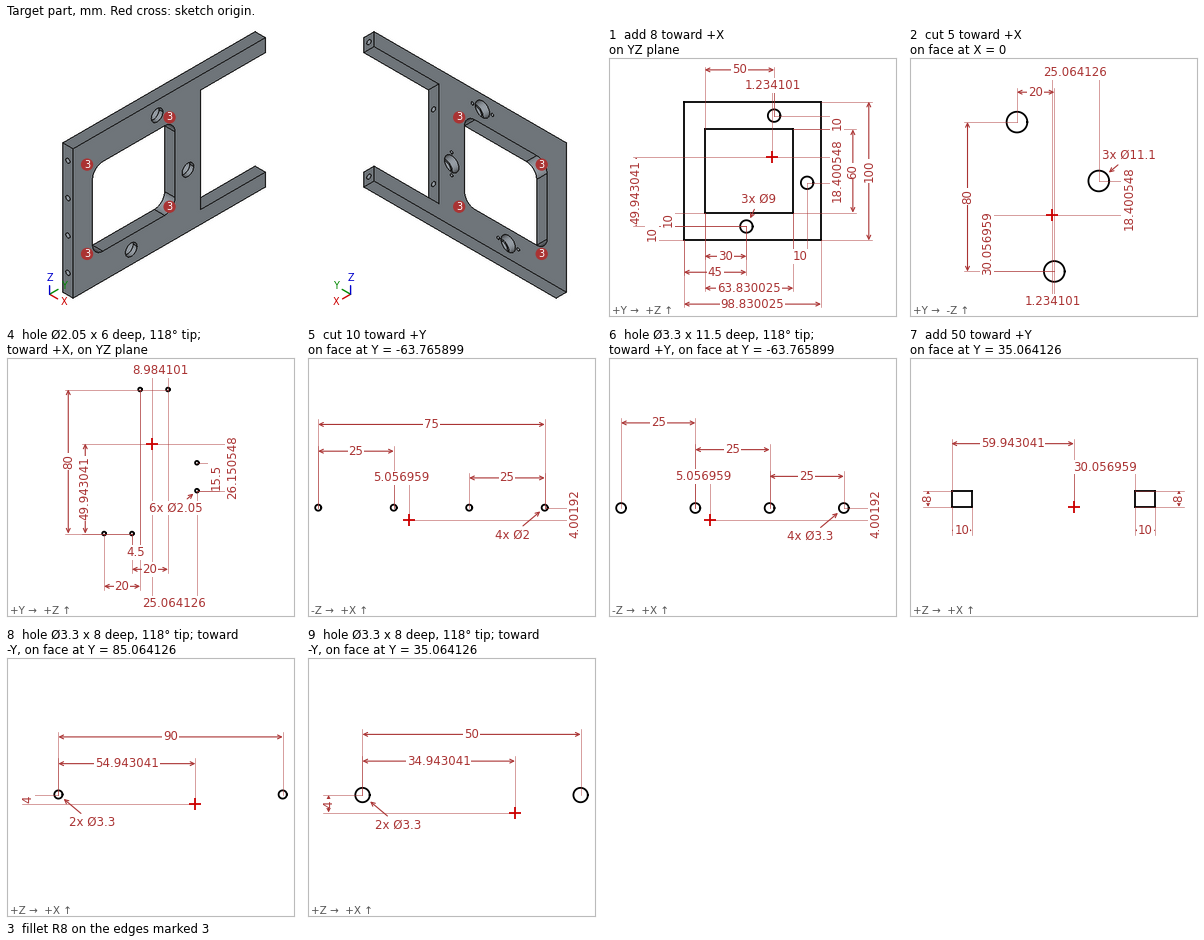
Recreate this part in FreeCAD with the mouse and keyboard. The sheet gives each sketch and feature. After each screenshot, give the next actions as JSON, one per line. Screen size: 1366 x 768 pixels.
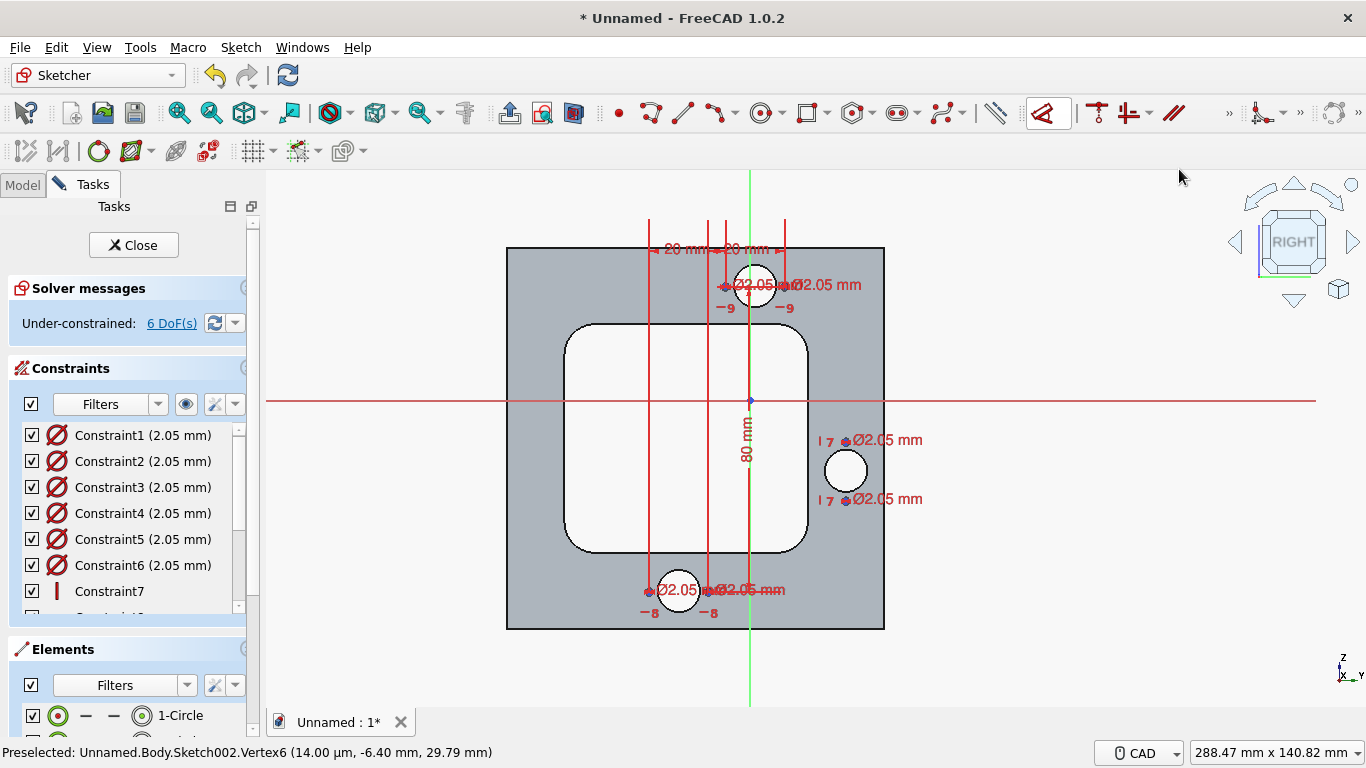
{"action": "scroll", "coordinate": [708, 592], "scroll_direction": "up", "scroll_amount": 5}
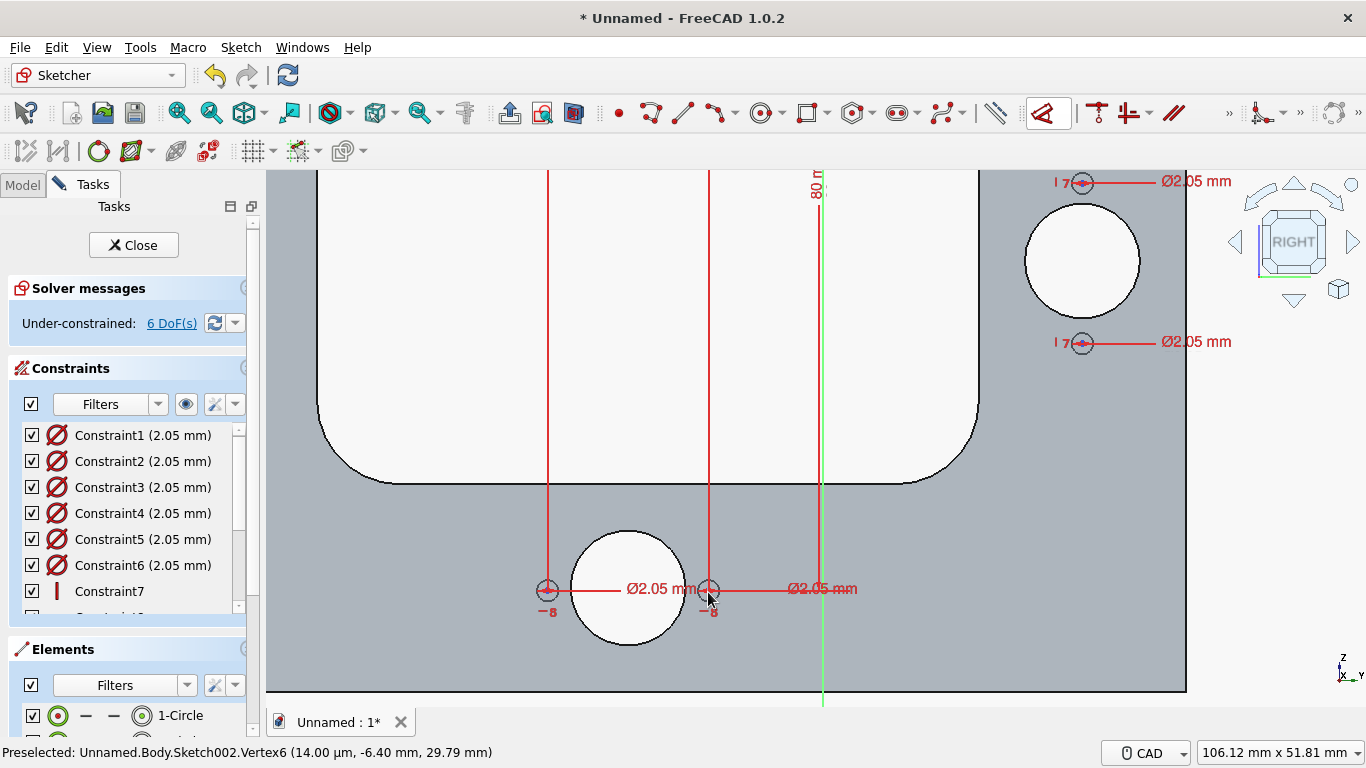
{"action": "left_click", "coordinate": [709, 591]}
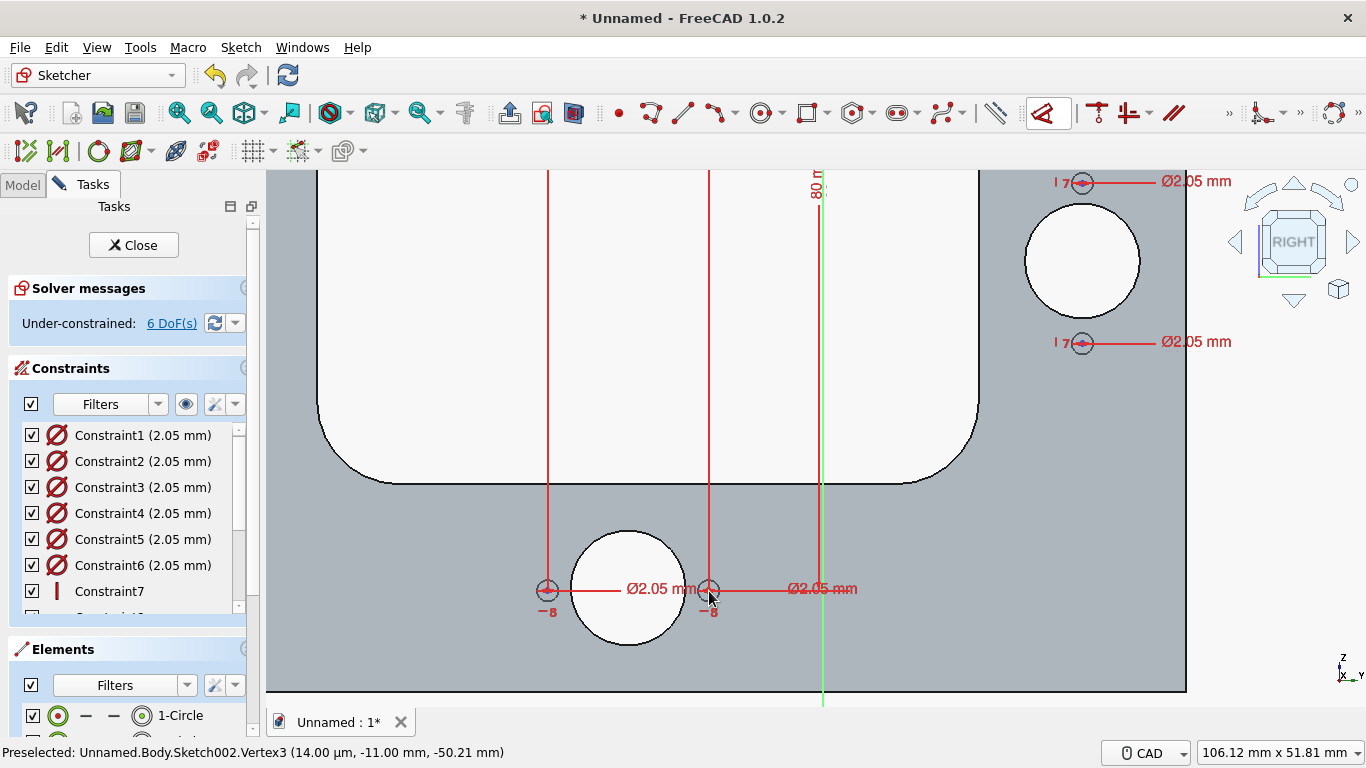
{"action": "scroll", "coordinate": [708, 593], "scroll_direction": "down", "scroll_amount": 5}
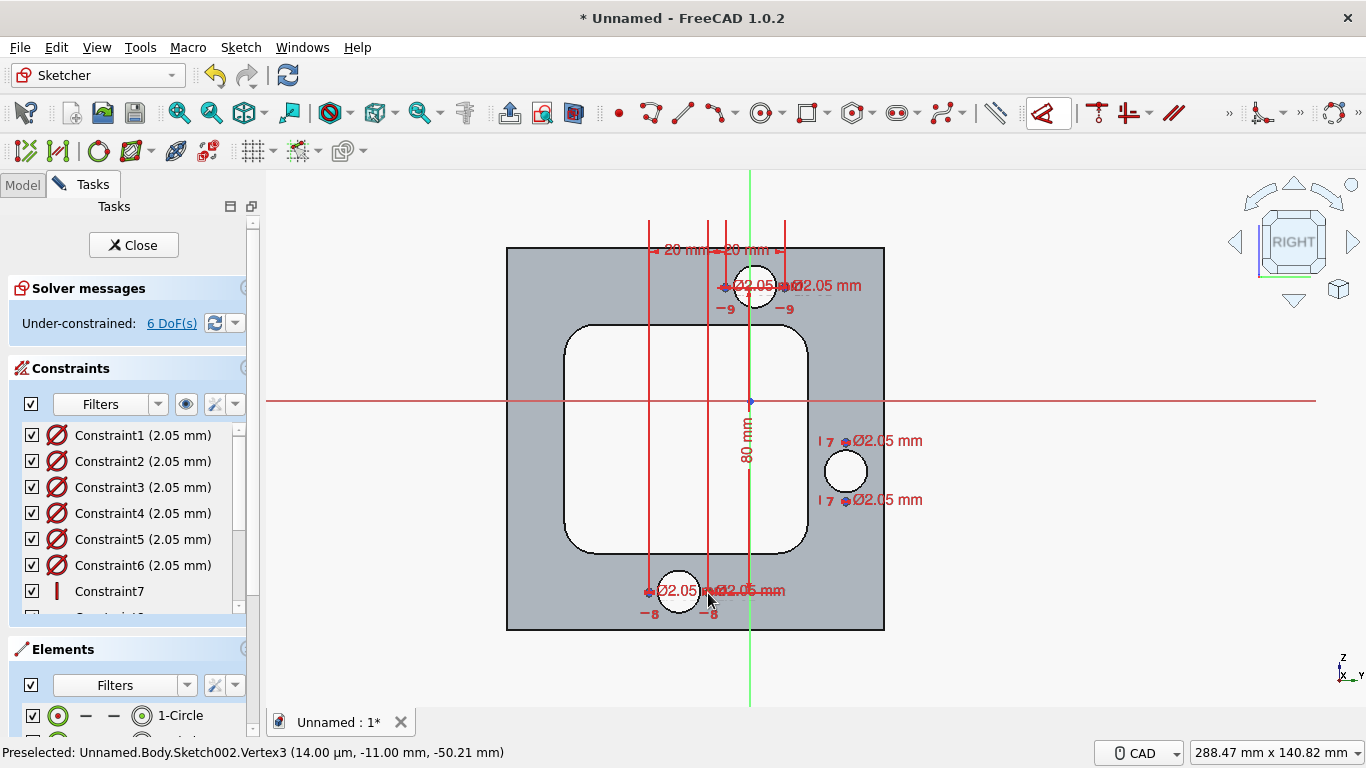
{"action": "scroll", "coordinate": [726, 288], "scroll_direction": "up", "scroll_amount": 5}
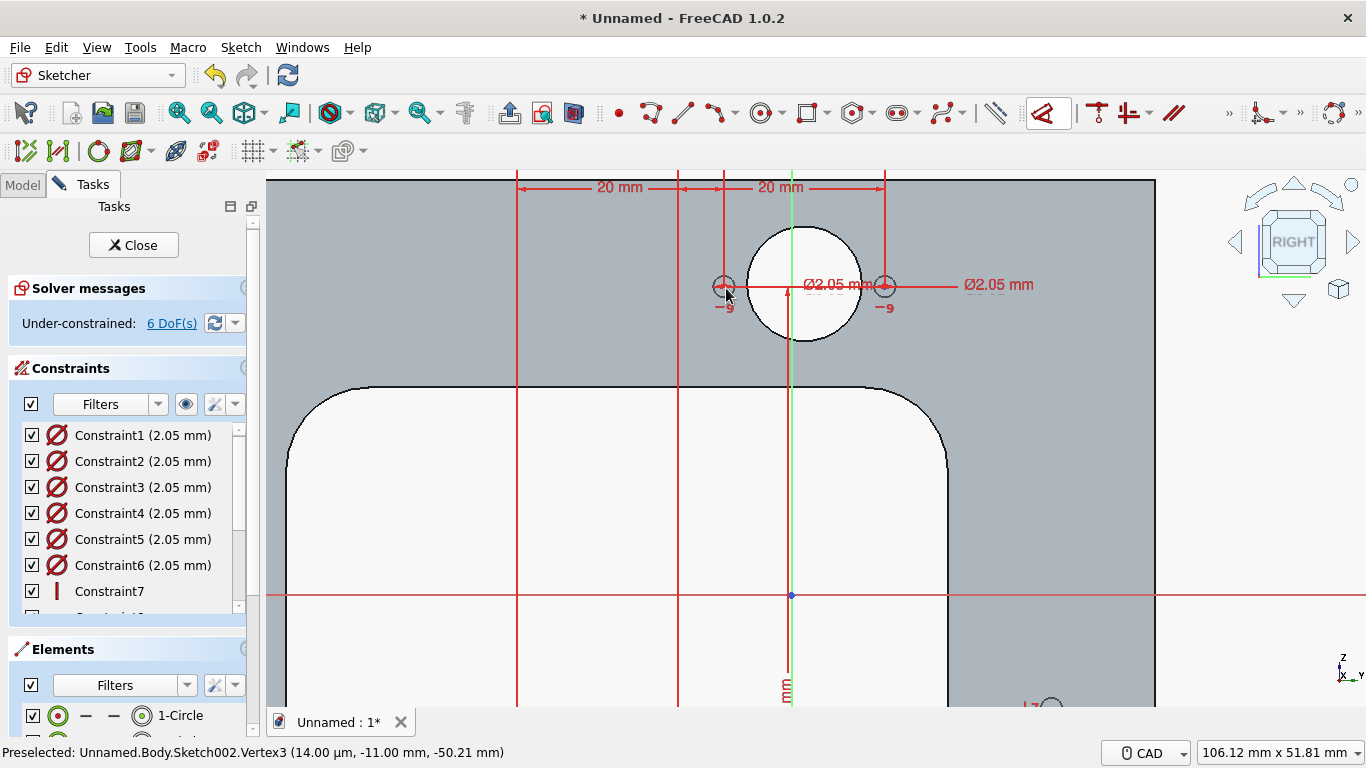
{"action": "left_click", "coordinate": [724, 287]}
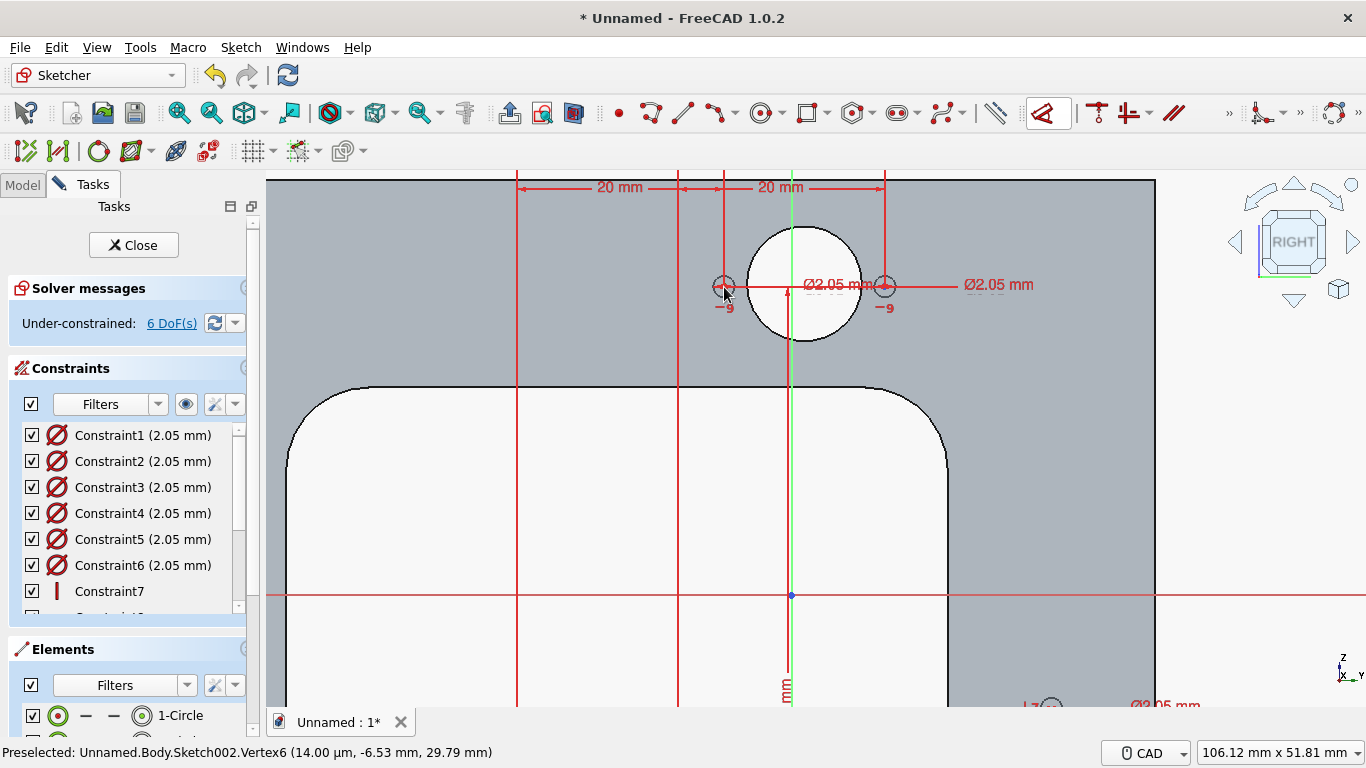
{"action": "key", "text": "l"}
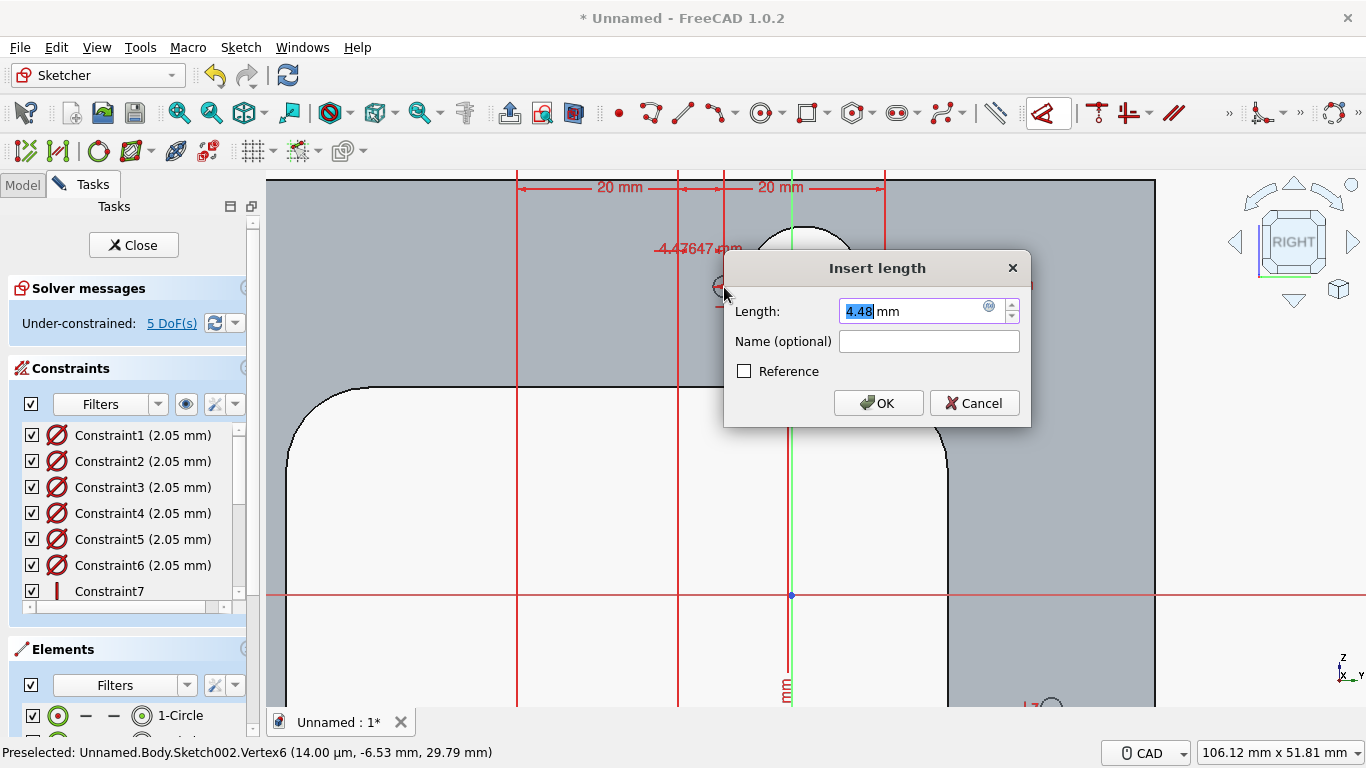
{"action": "type", "text": "4.5"}
{"action": "key", "text": "Return"}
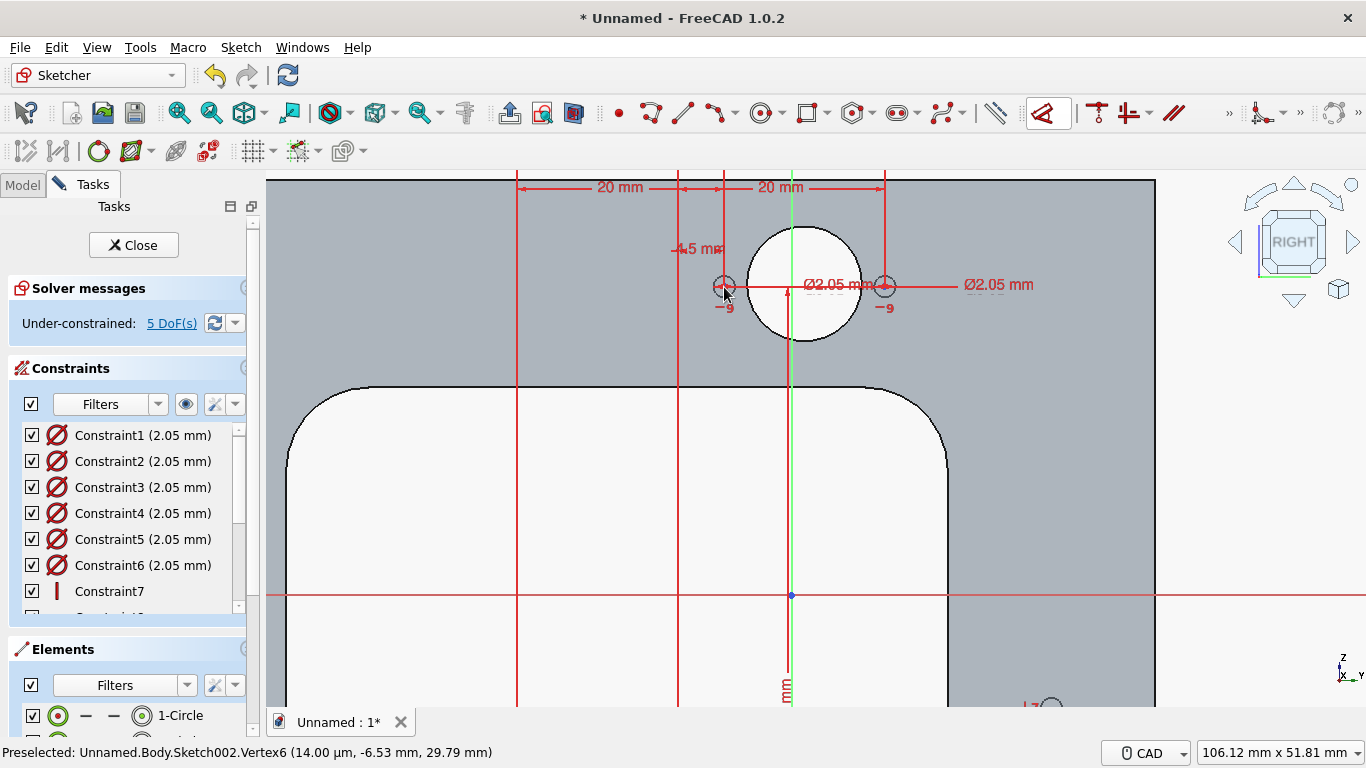
{"action": "scroll", "coordinate": [726, 287], "scroll_direction": "down", "scroll_amount": 5}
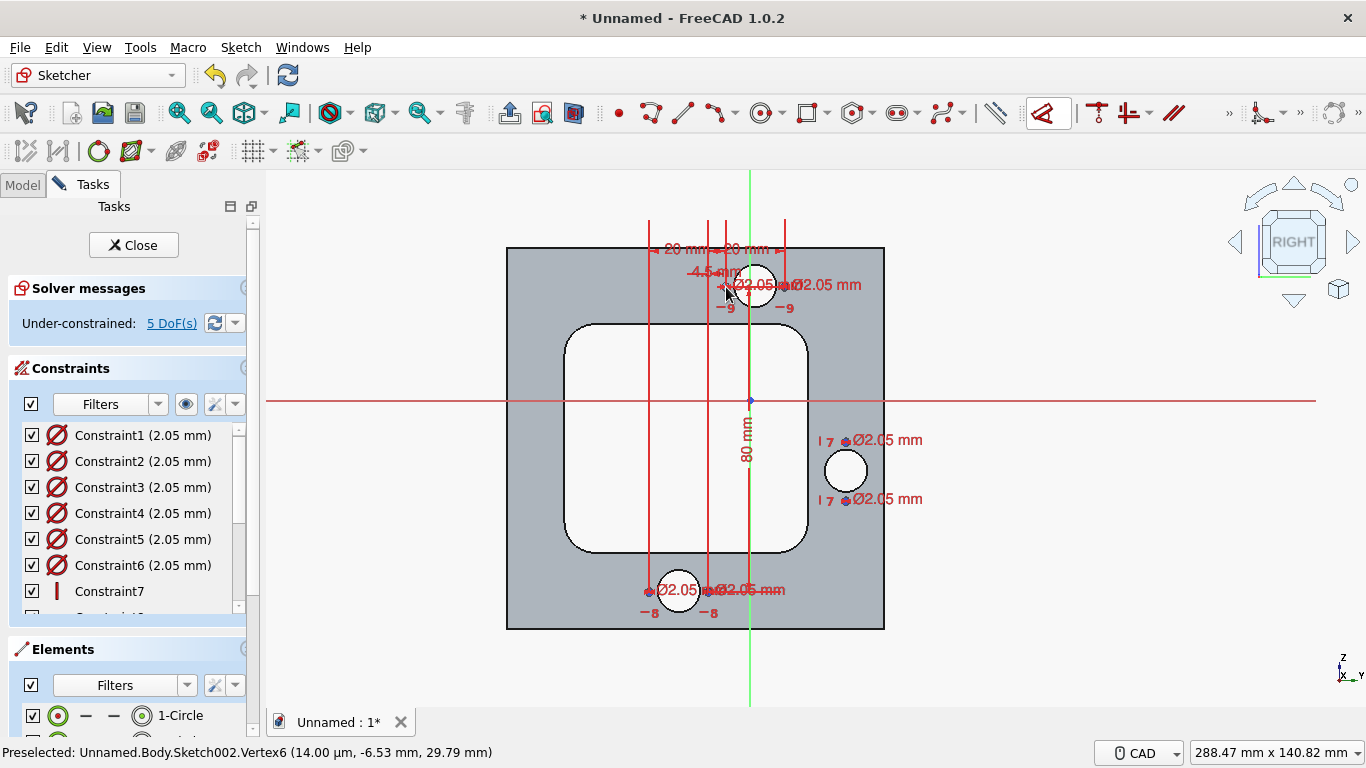
{"action": "left_click", "coordinate": [846, 501]}